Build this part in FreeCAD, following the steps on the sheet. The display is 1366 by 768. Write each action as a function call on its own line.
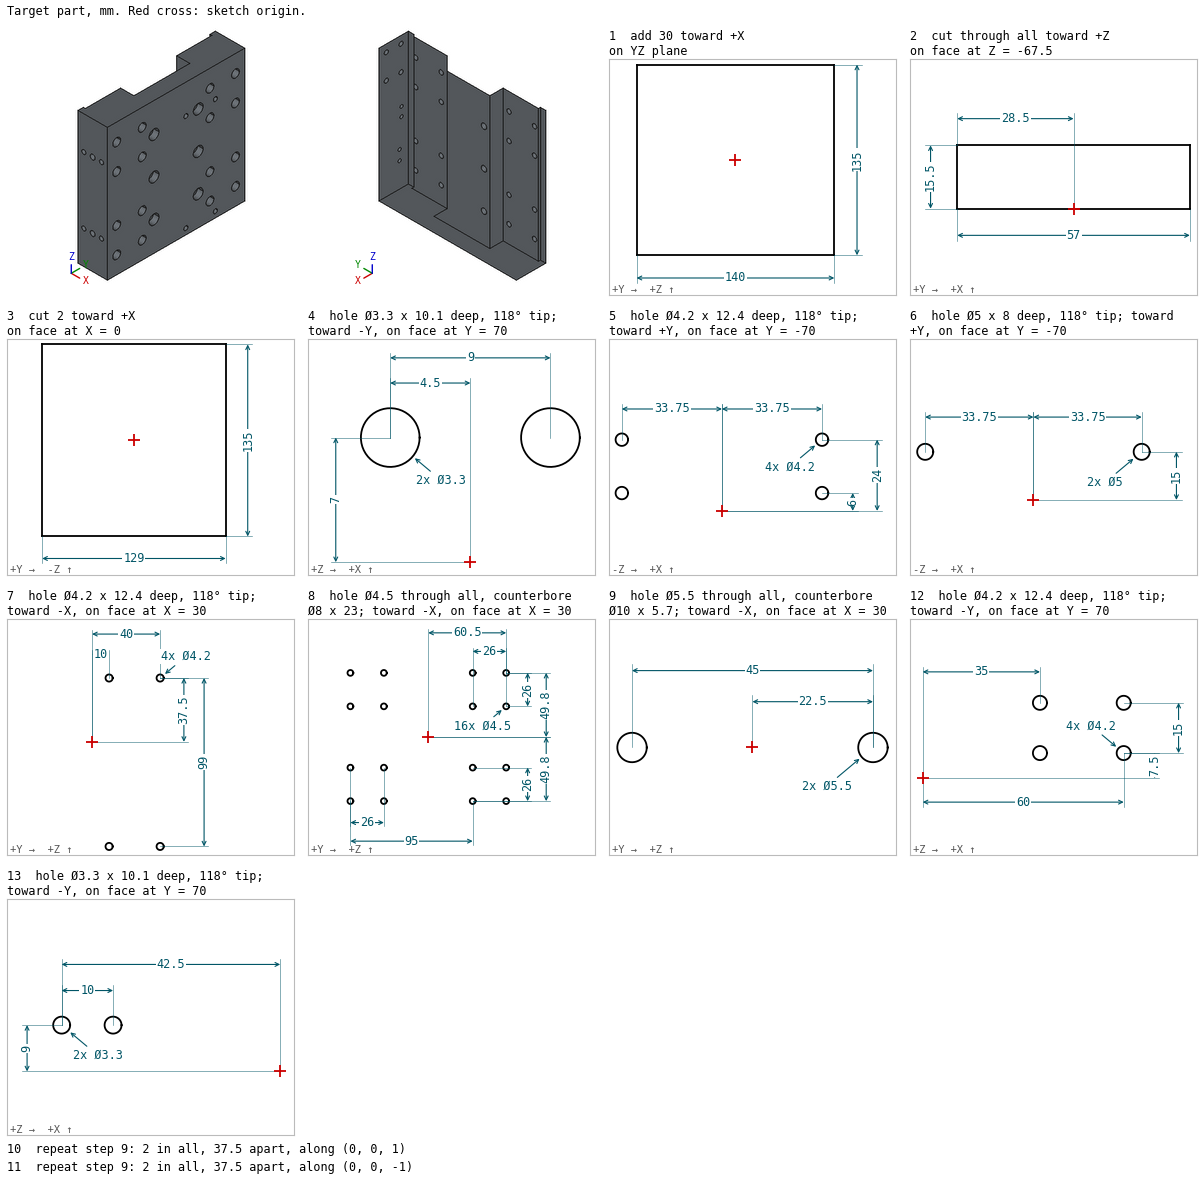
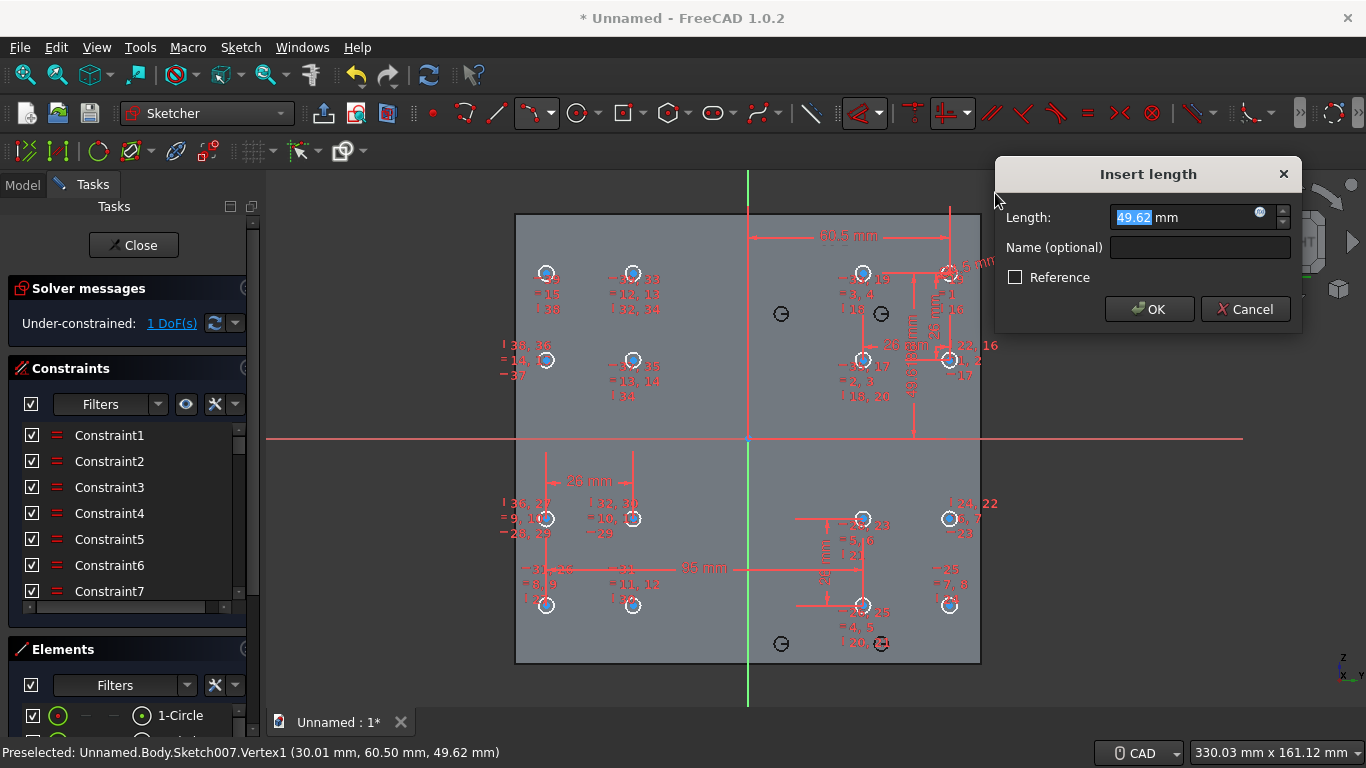
text(49.8)
key(Return)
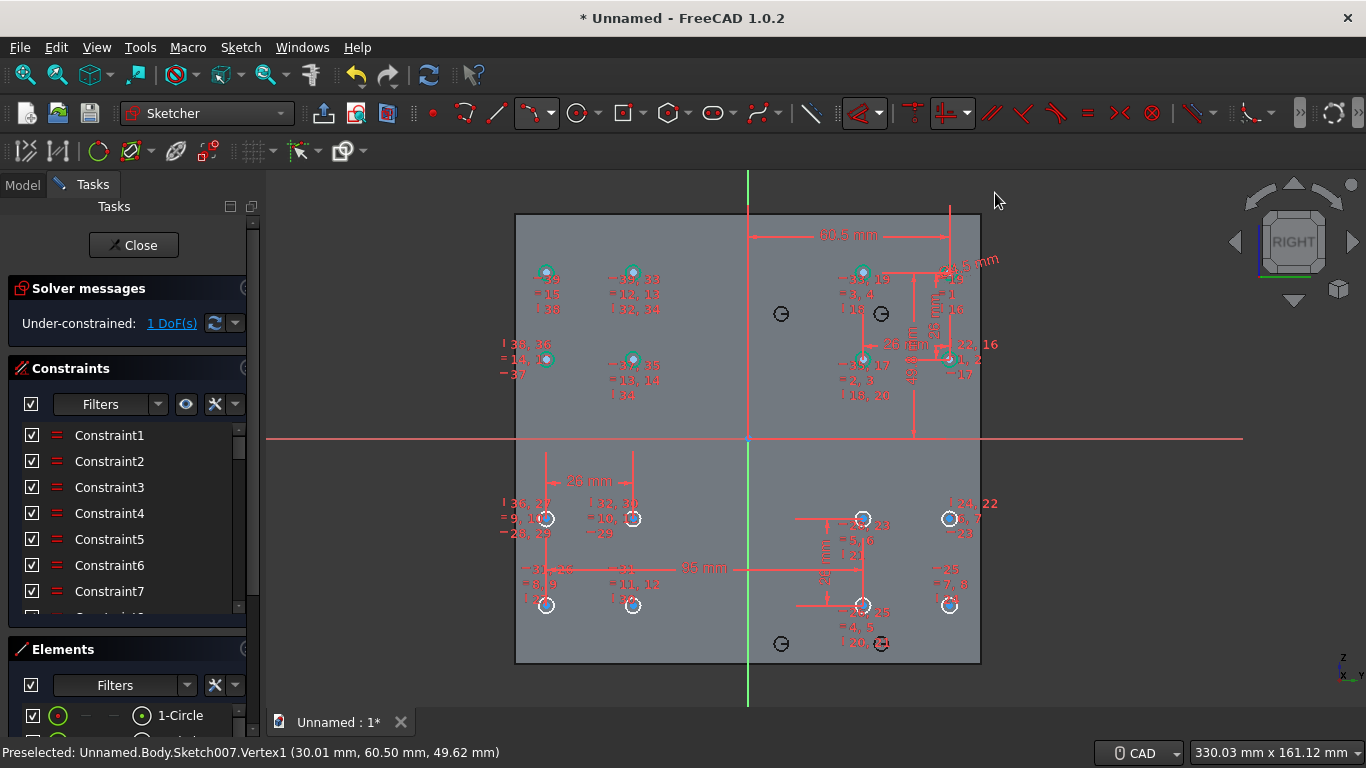
click(863, 606)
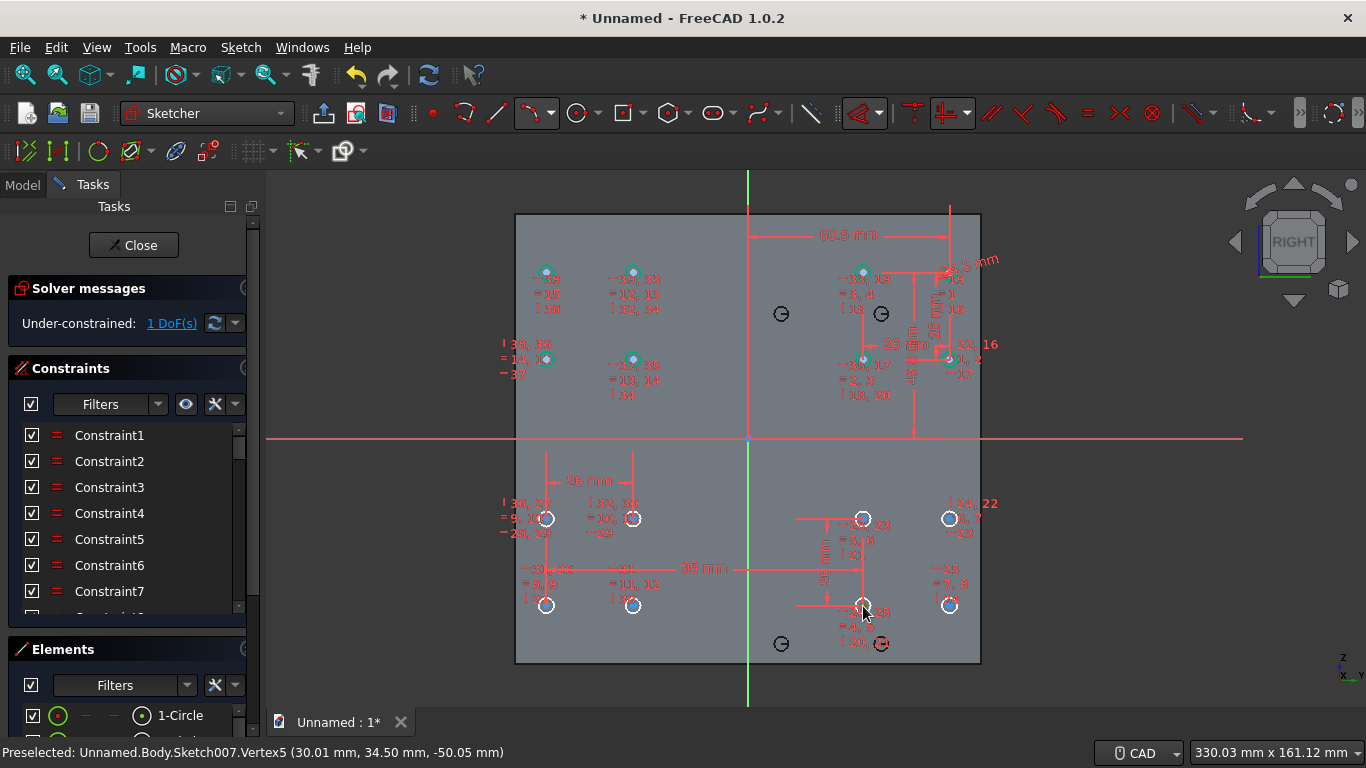
key(i)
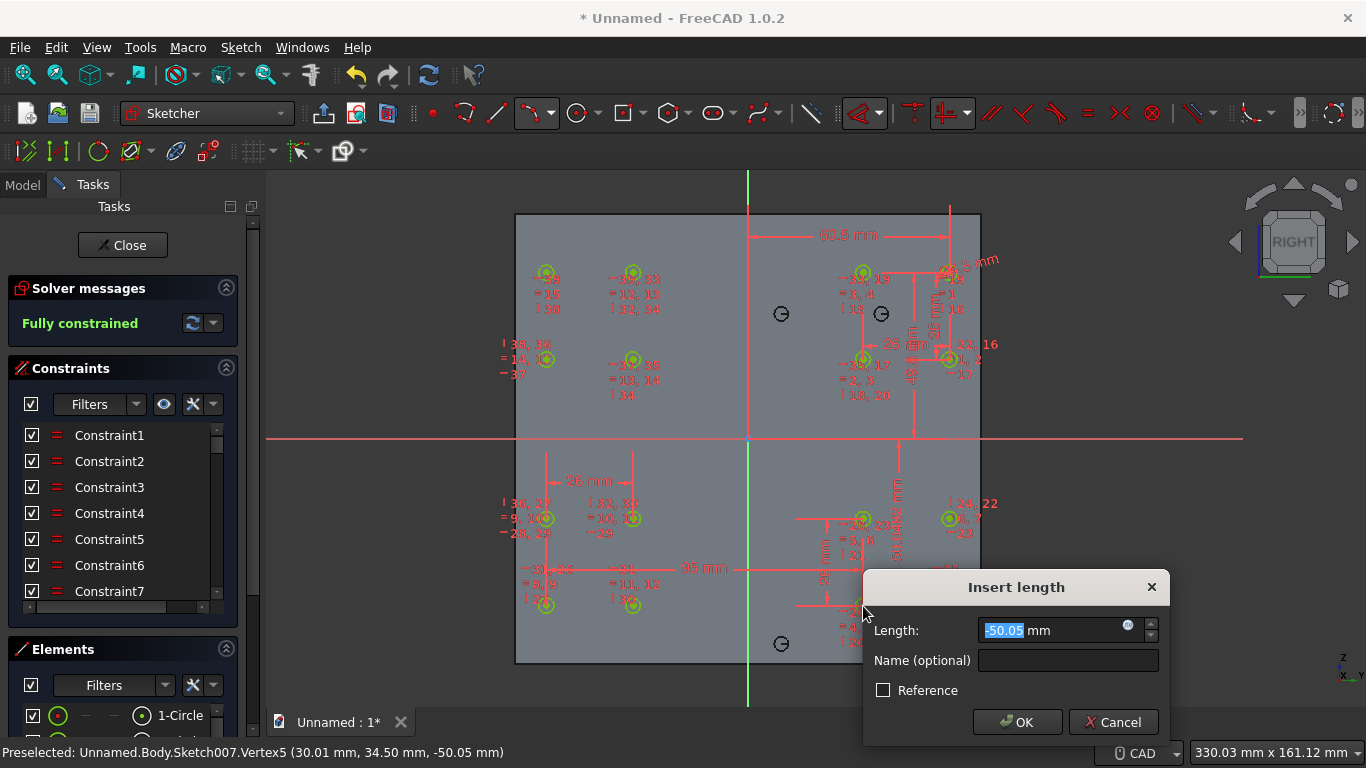
text(-49.8)
key(Return)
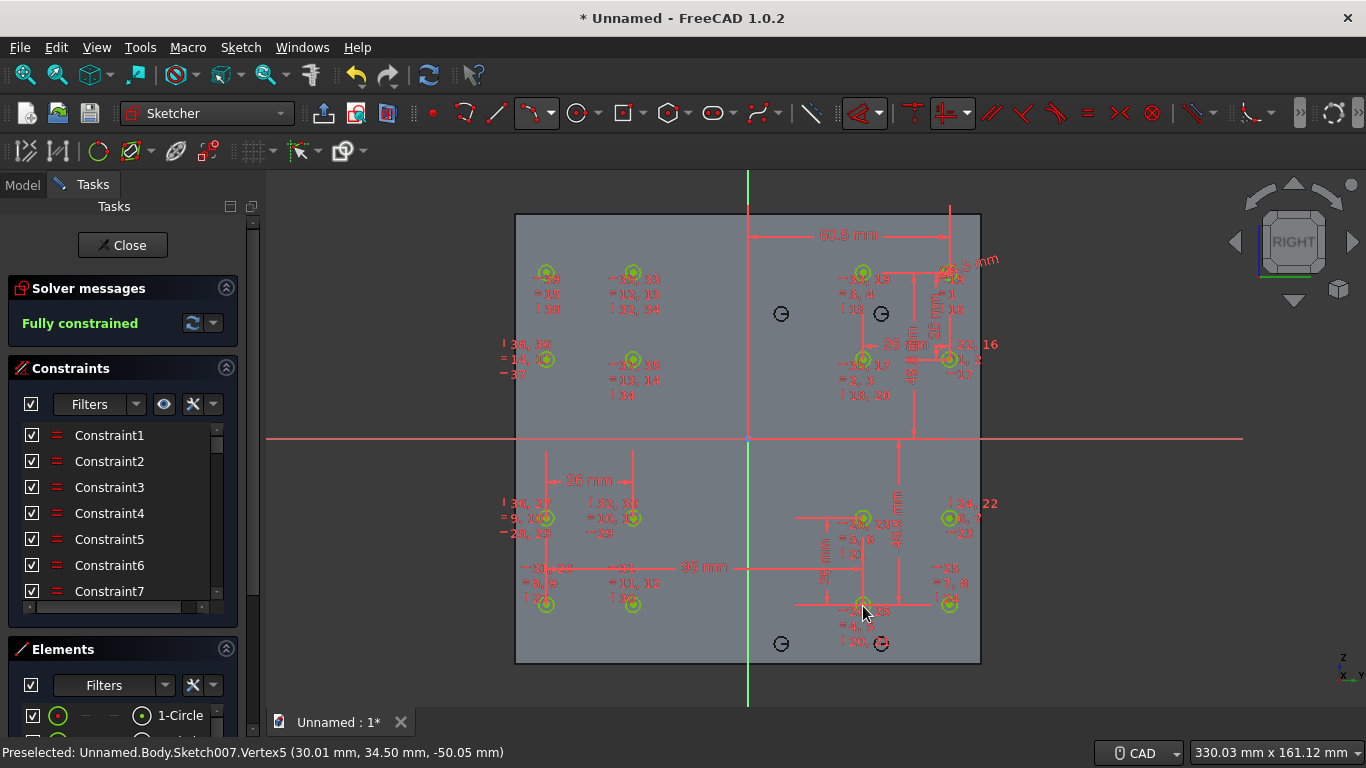
click(123, 245)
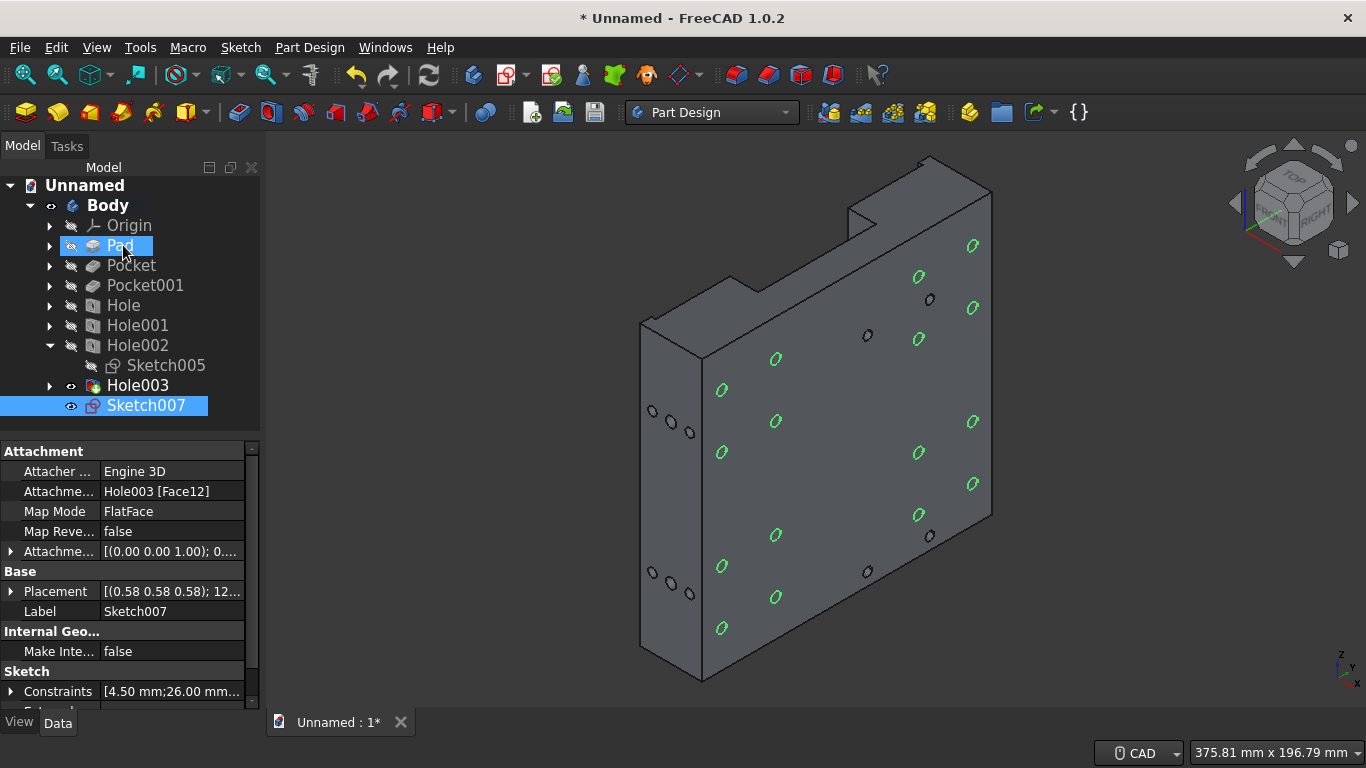
click(272, 112)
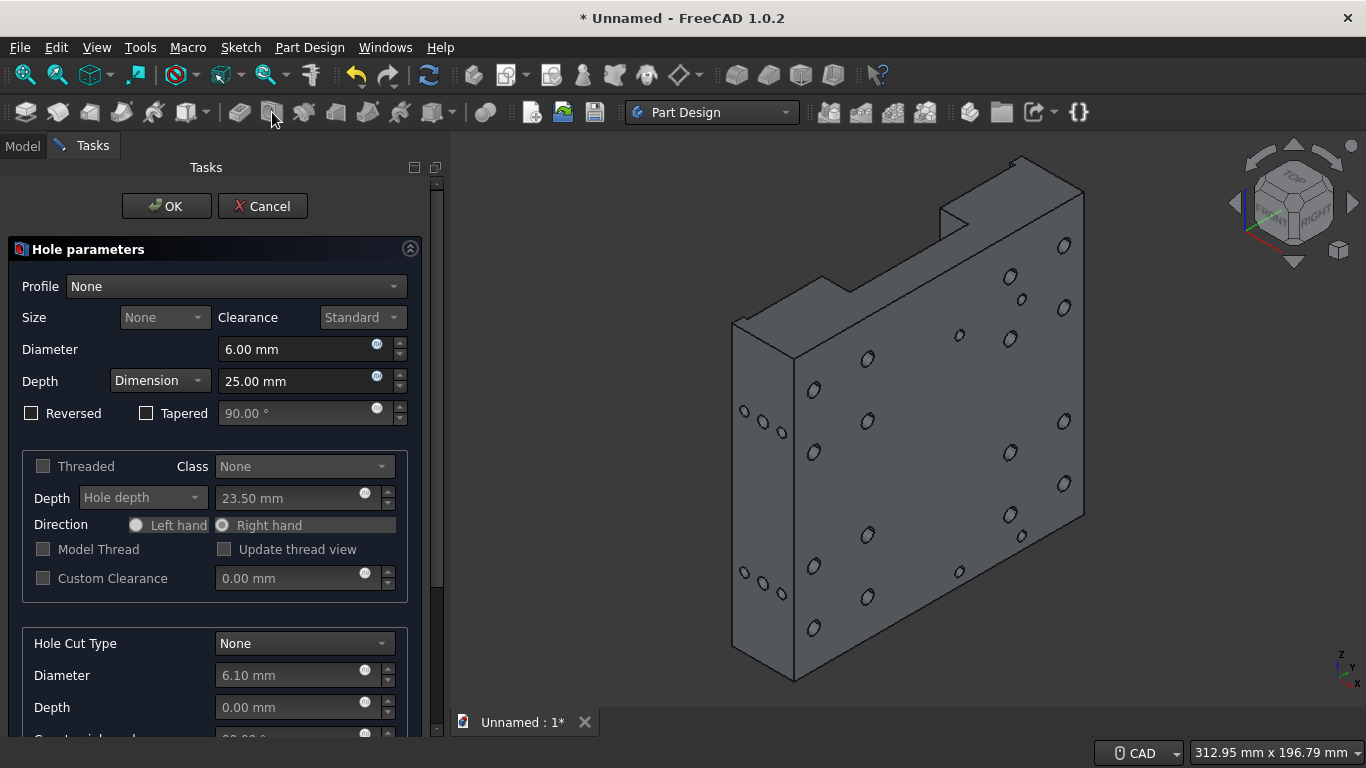
triple_click(305, 349)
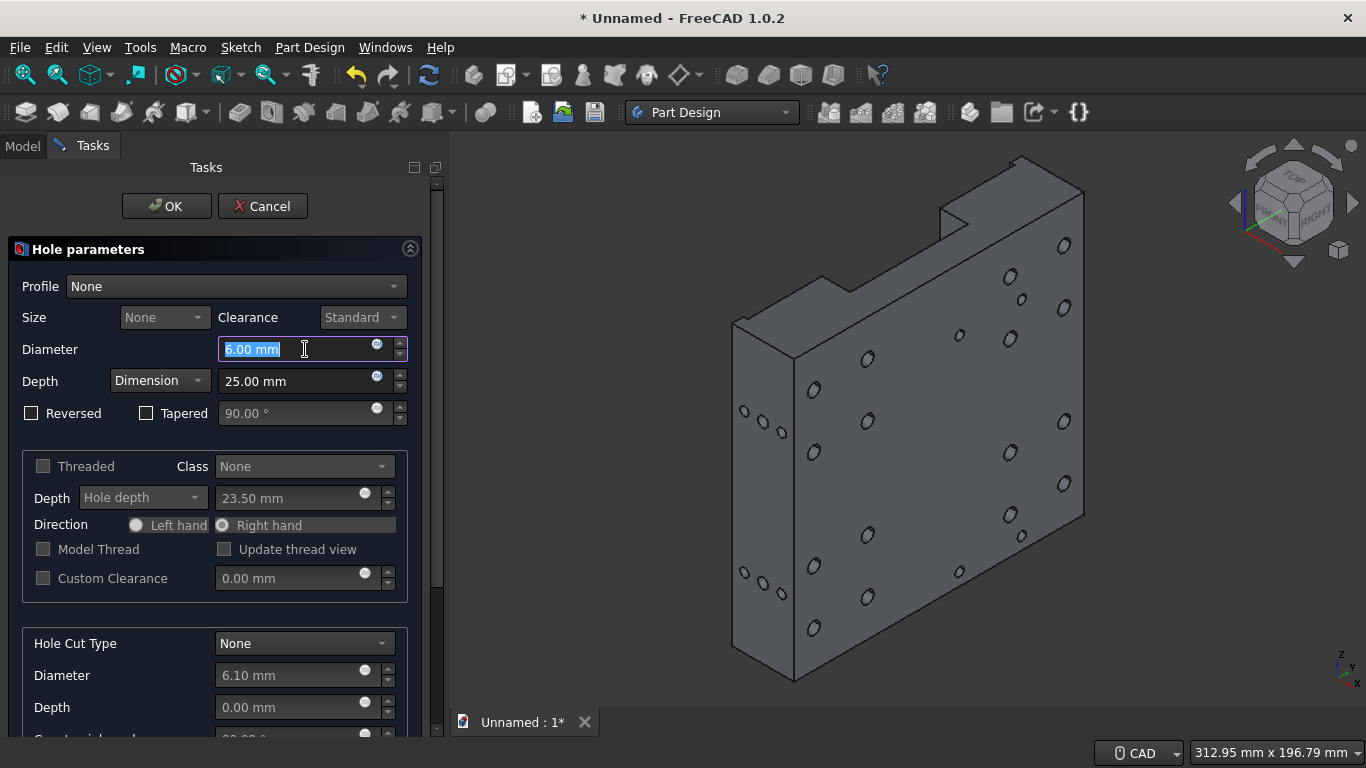
text(4.5)
key(Tab)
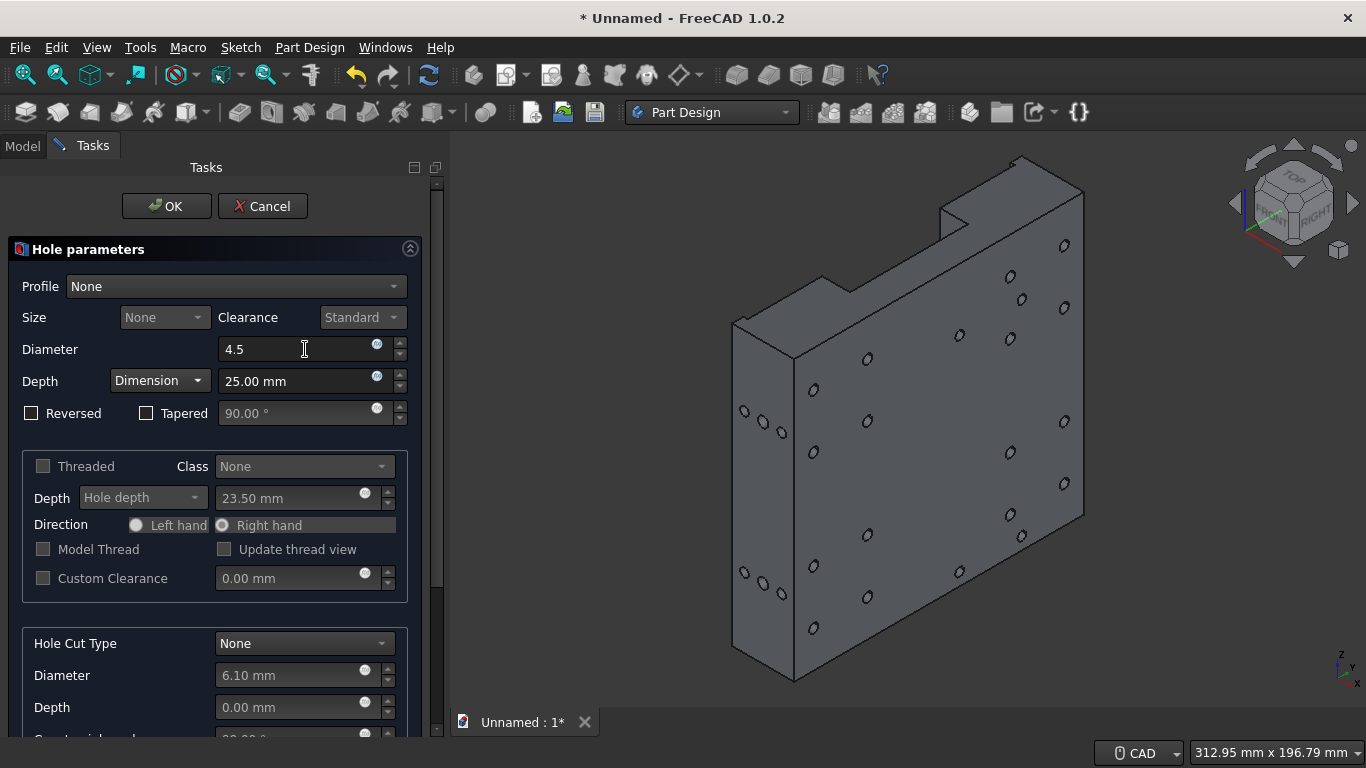
click(161, 380)